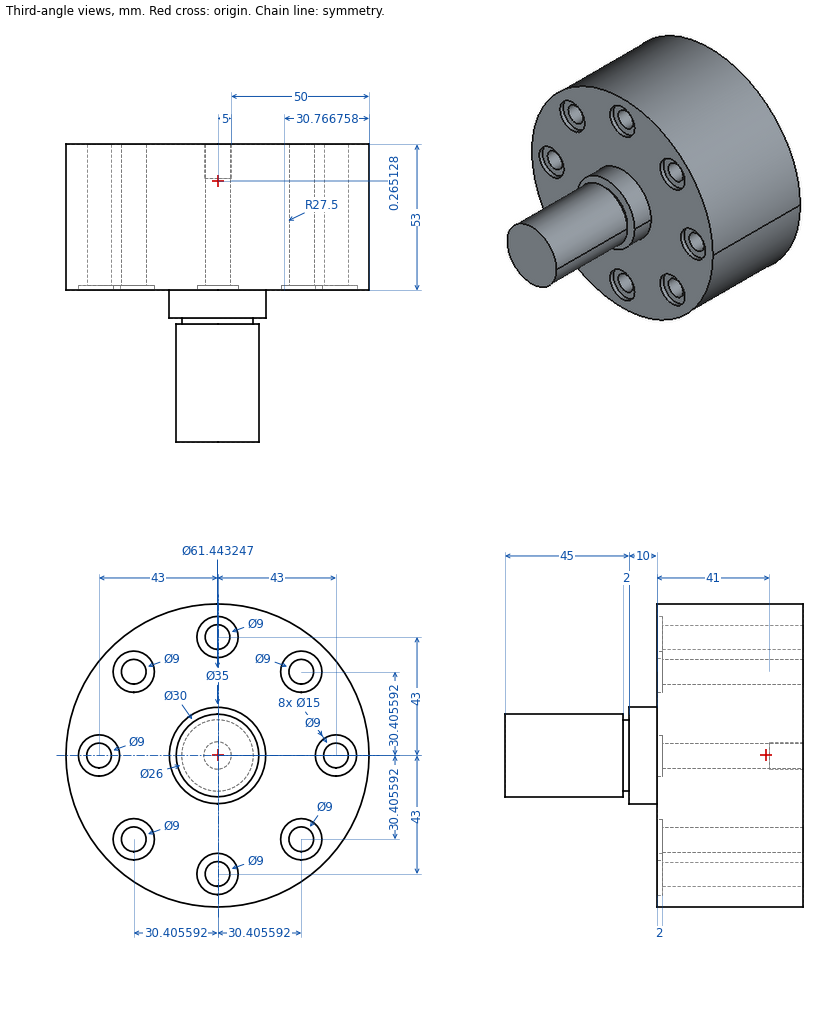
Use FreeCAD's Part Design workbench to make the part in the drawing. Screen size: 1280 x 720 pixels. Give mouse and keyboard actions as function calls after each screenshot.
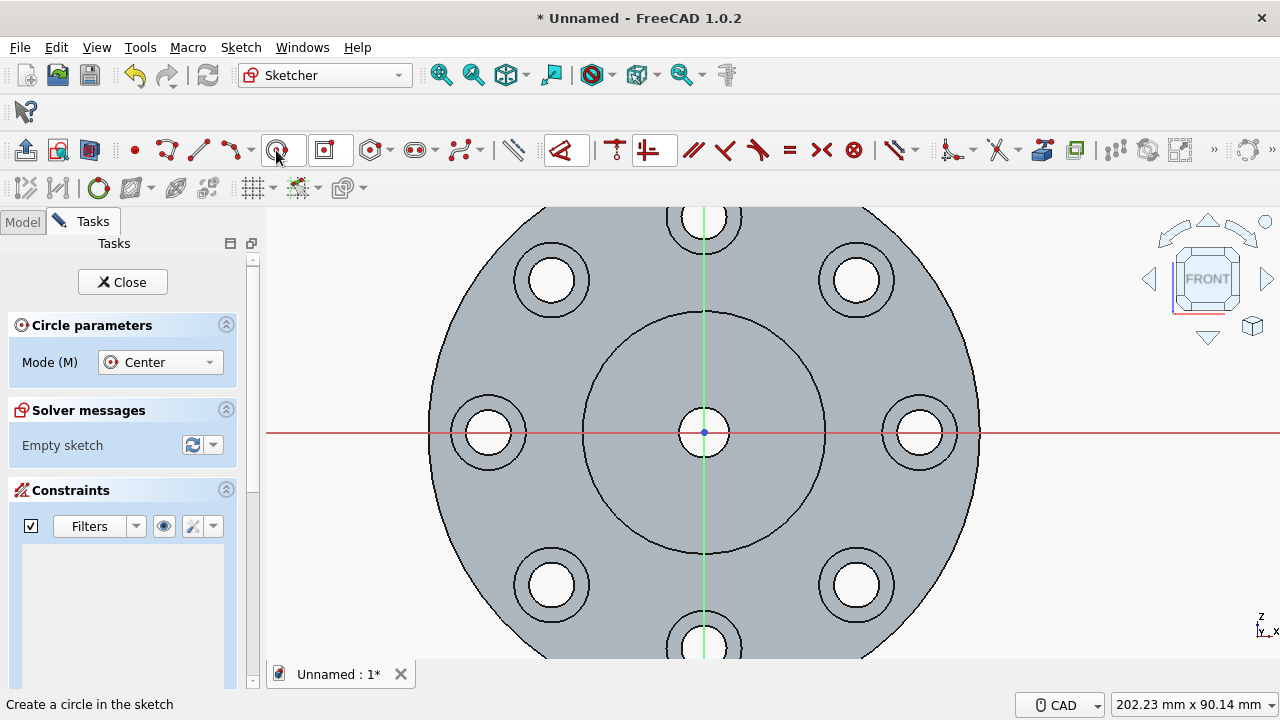
click(704, 433)
move(813, 324)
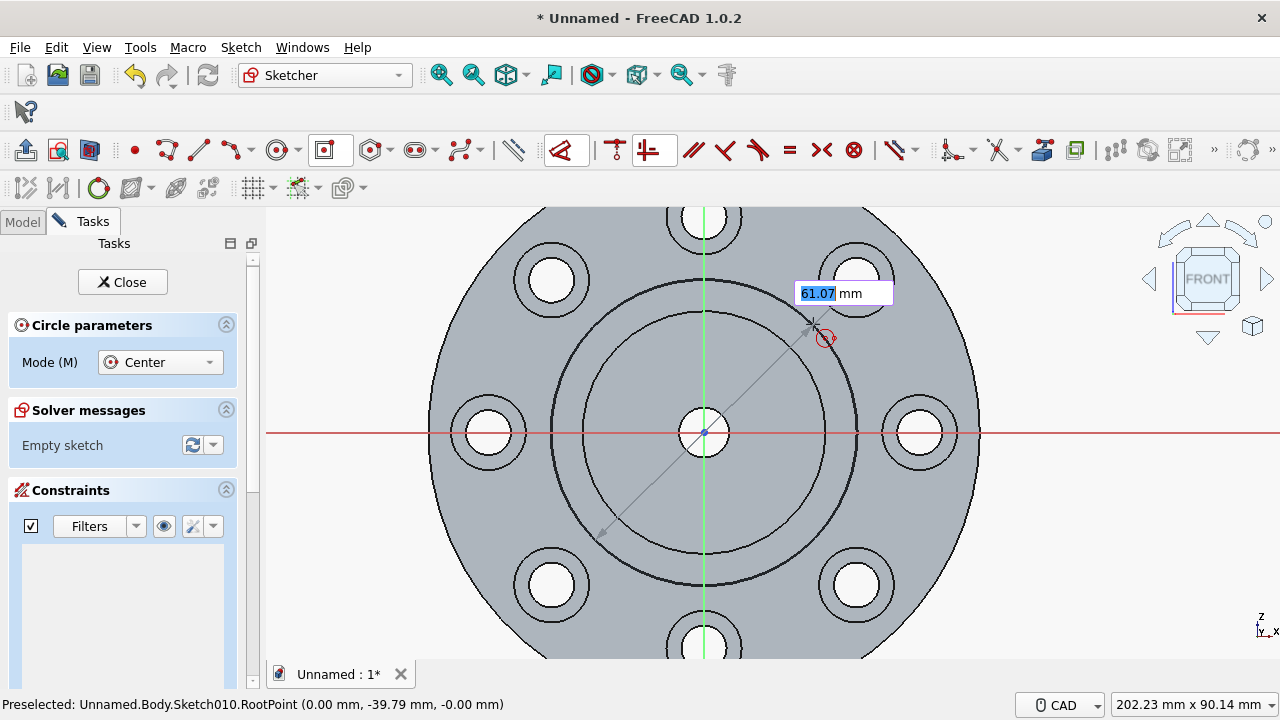
text(61.443247)
key(Return)
key(Escape)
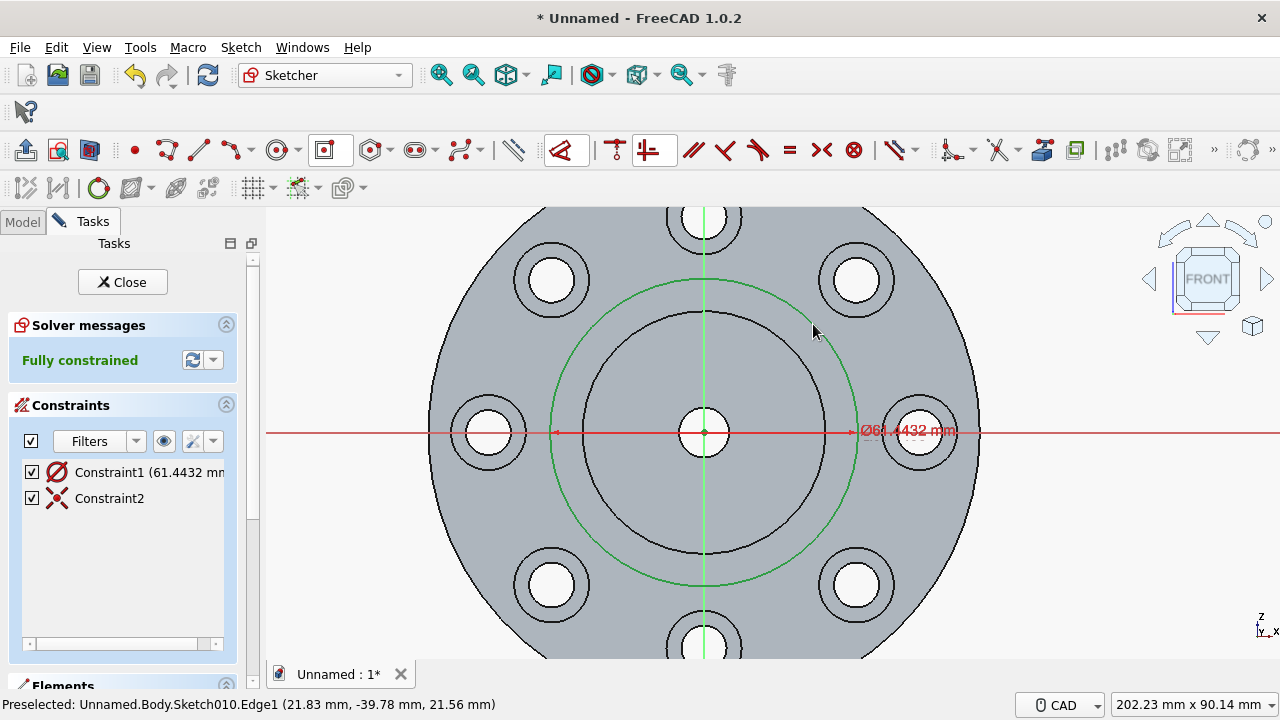
click(123, 282)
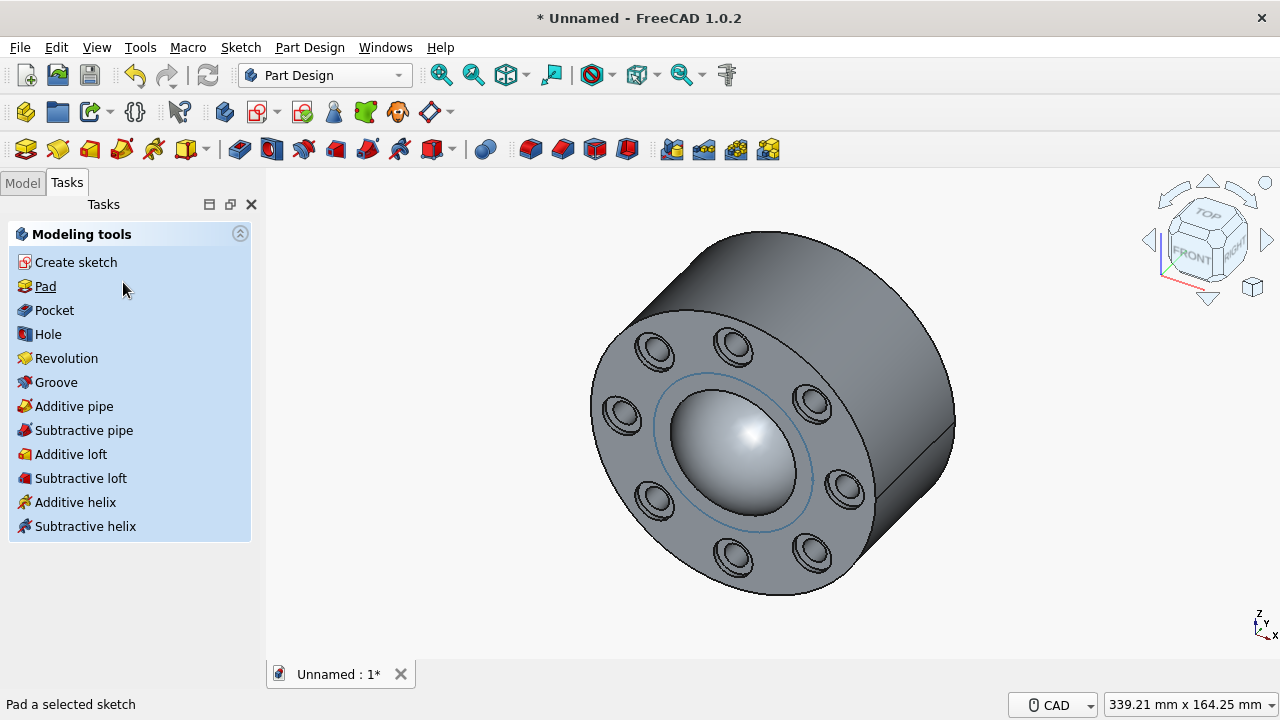
click(26, 150)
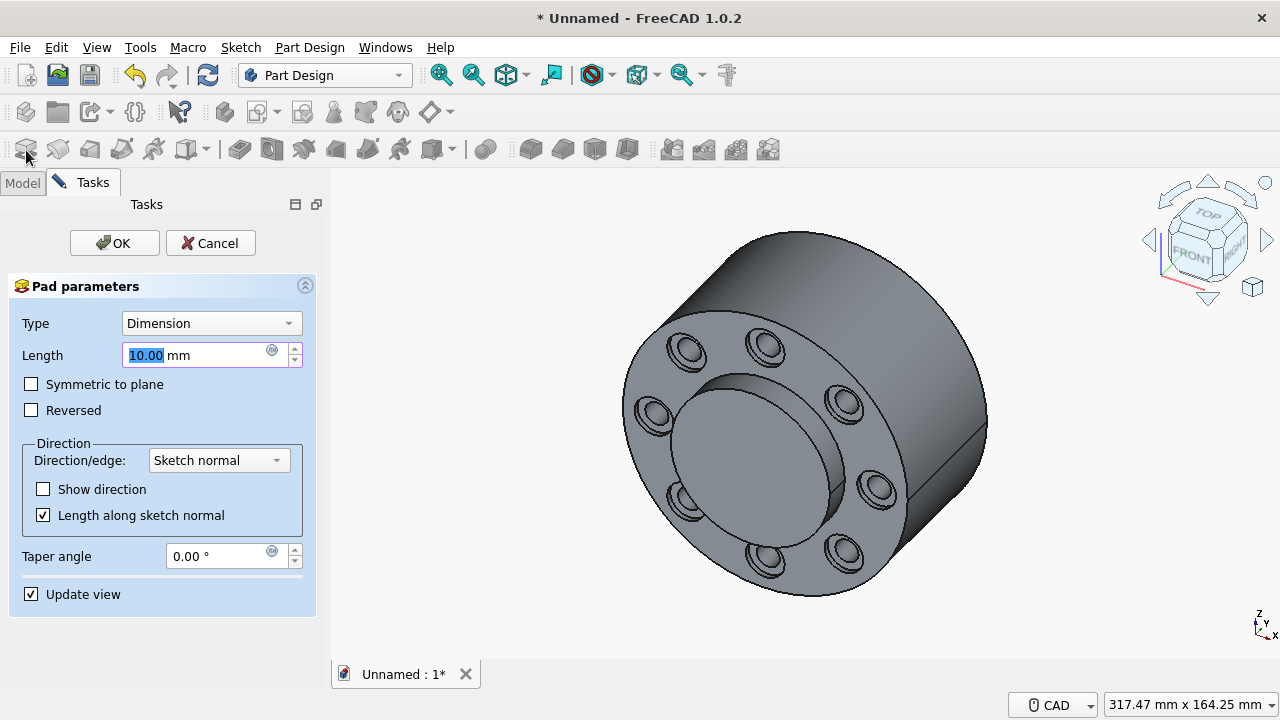
text(41)
key(Tab)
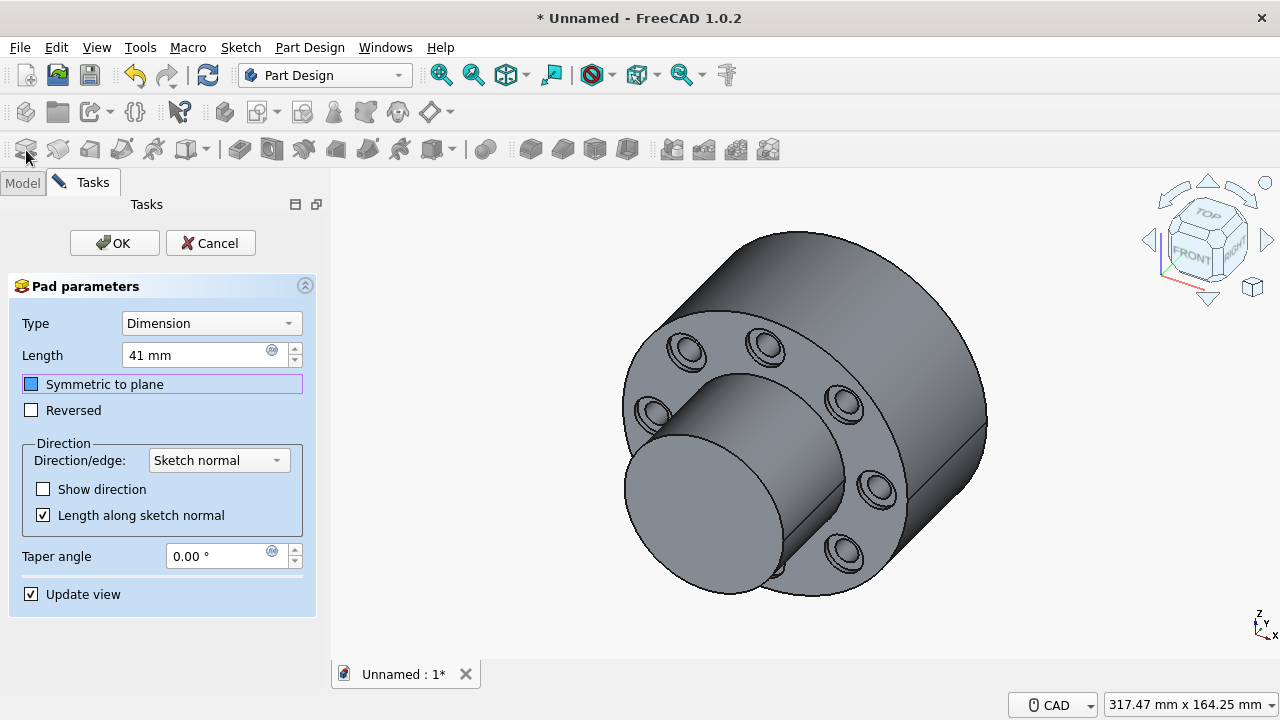
click(30, 410)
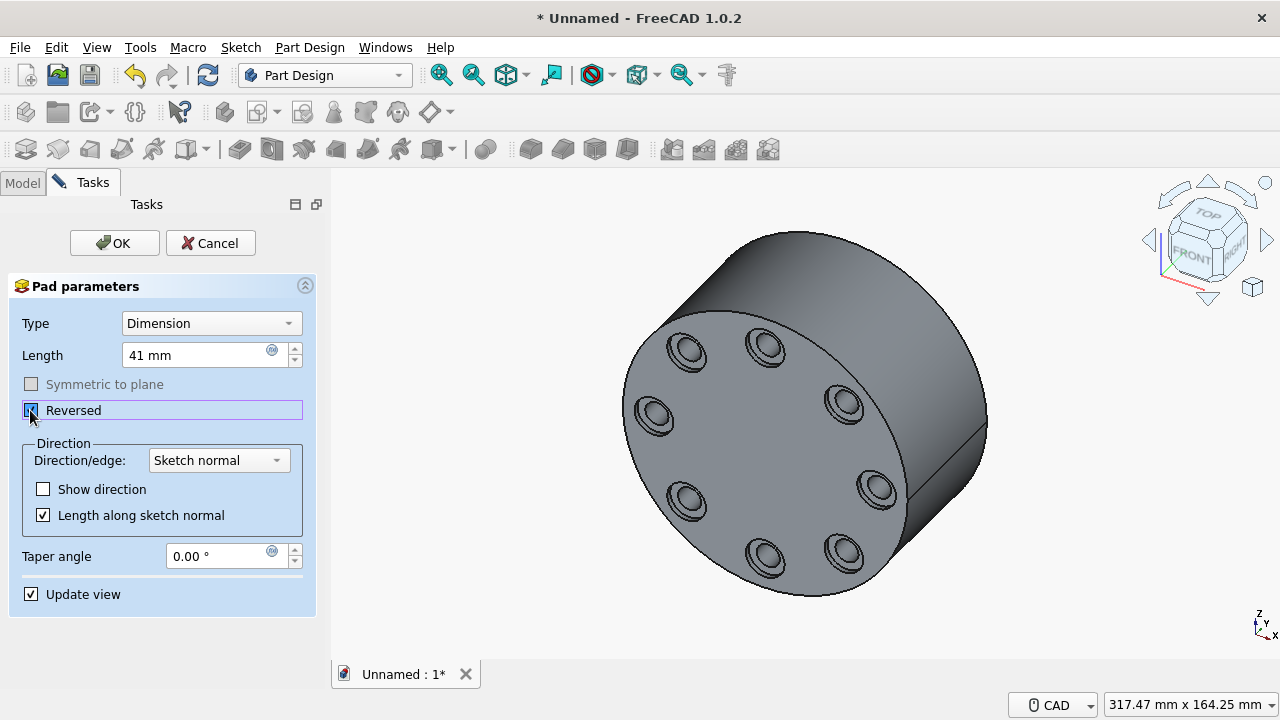
click(115, 243)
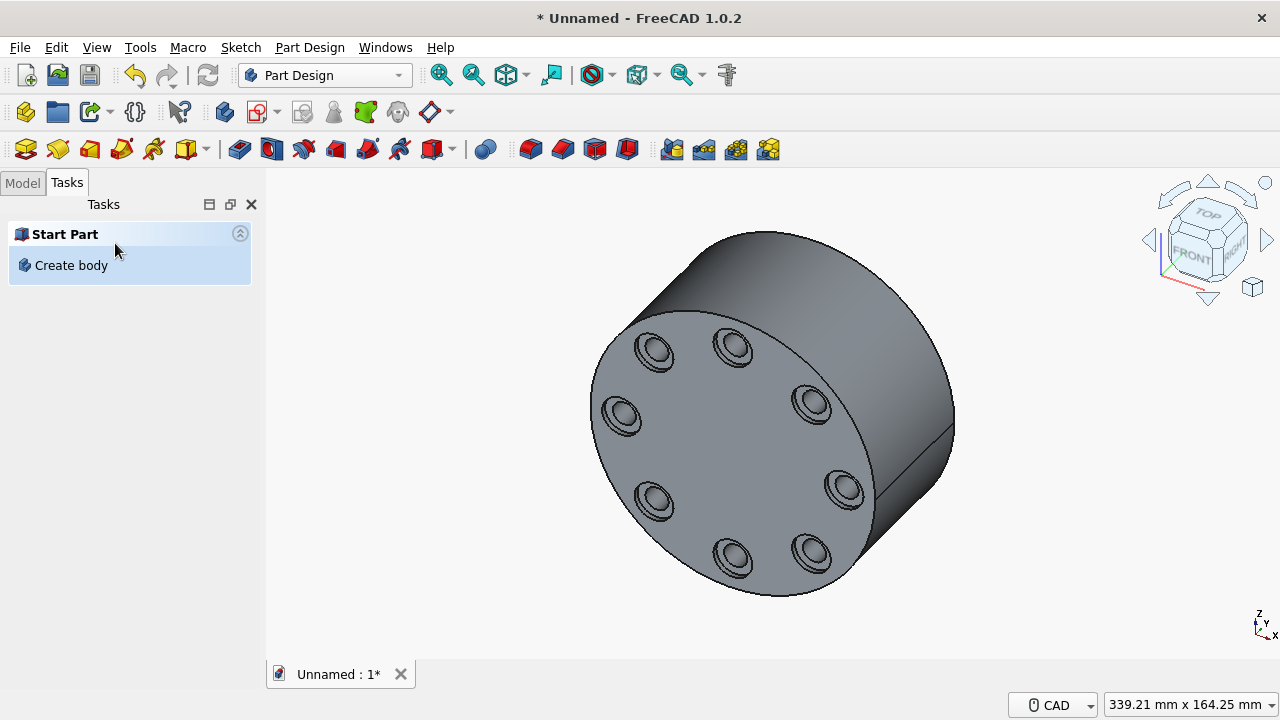
click(733, 452)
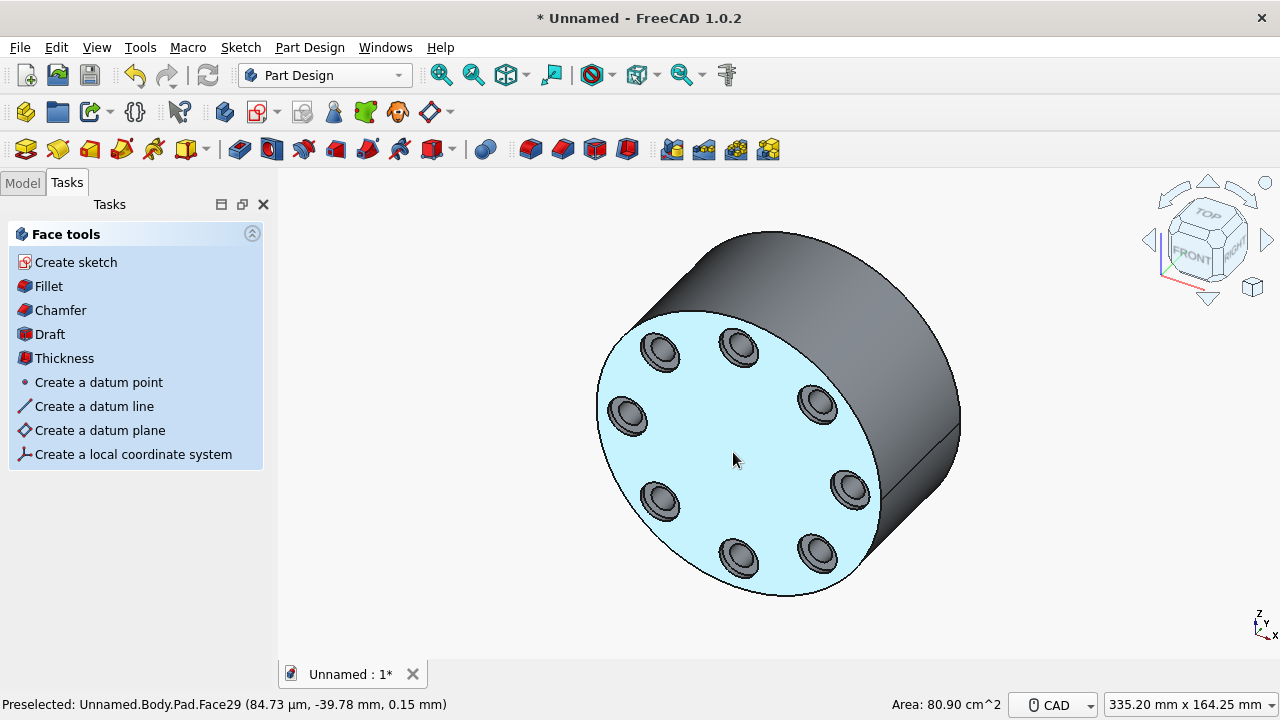
click(258, 112)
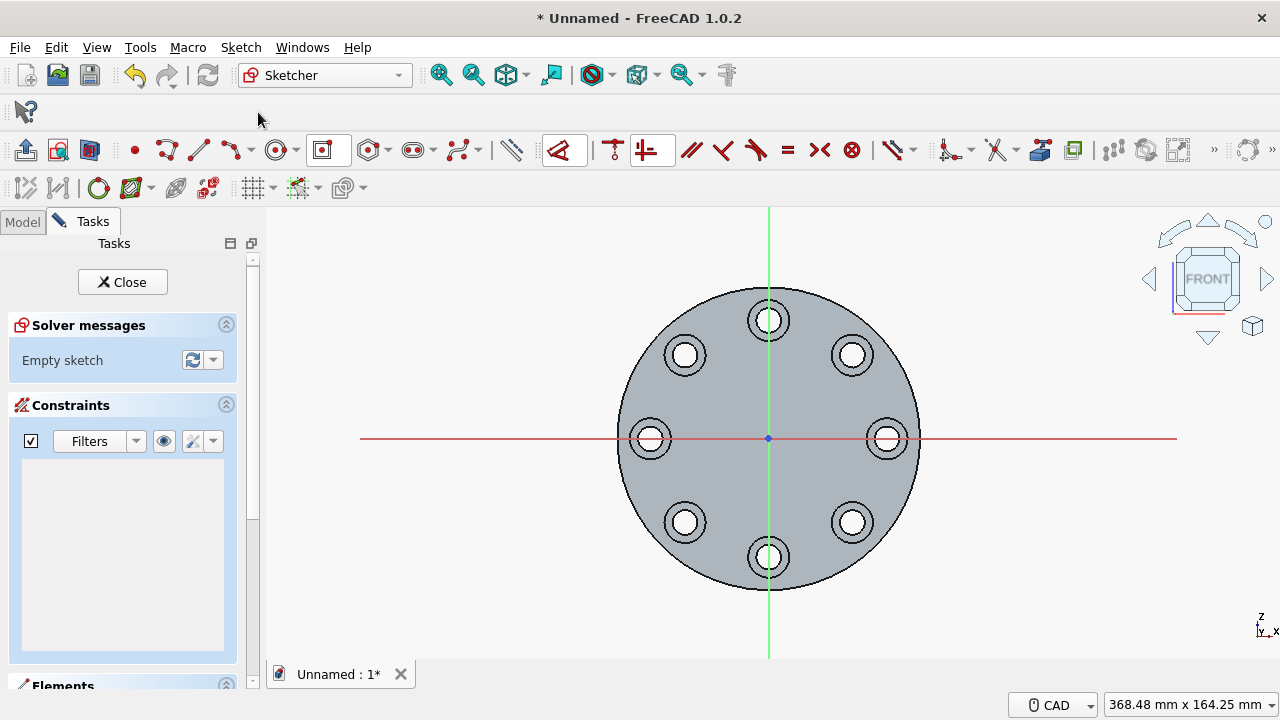
scroll(806, 442, up, 5)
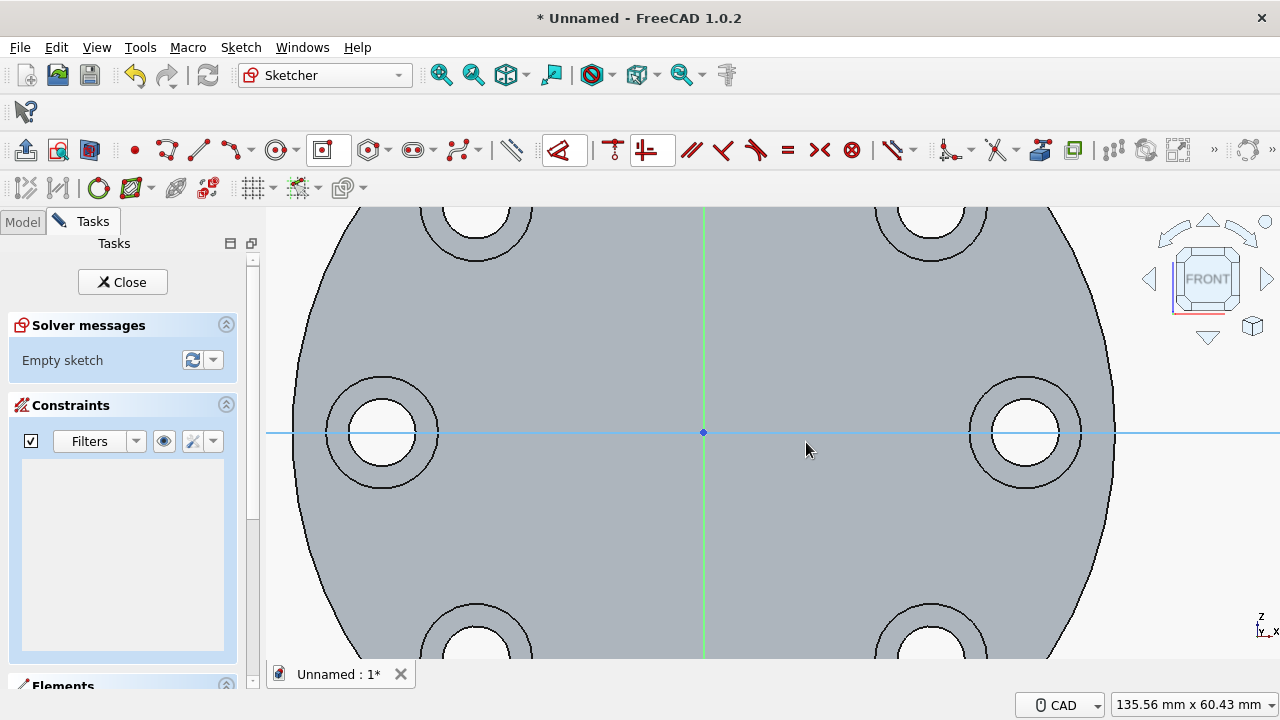
click(276, 150)